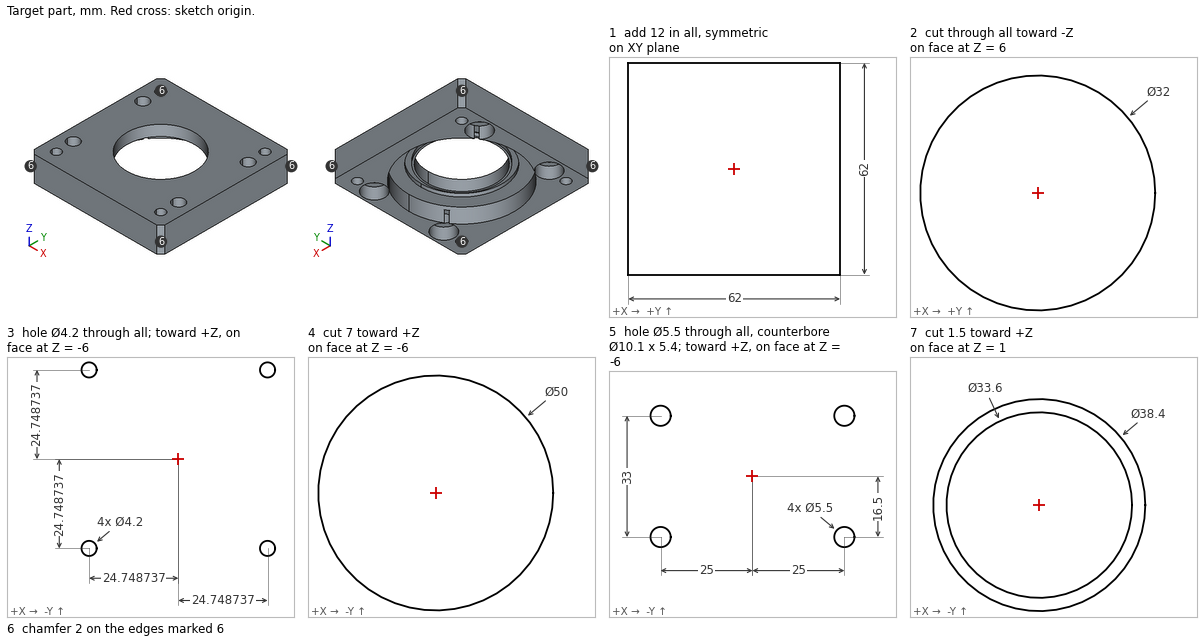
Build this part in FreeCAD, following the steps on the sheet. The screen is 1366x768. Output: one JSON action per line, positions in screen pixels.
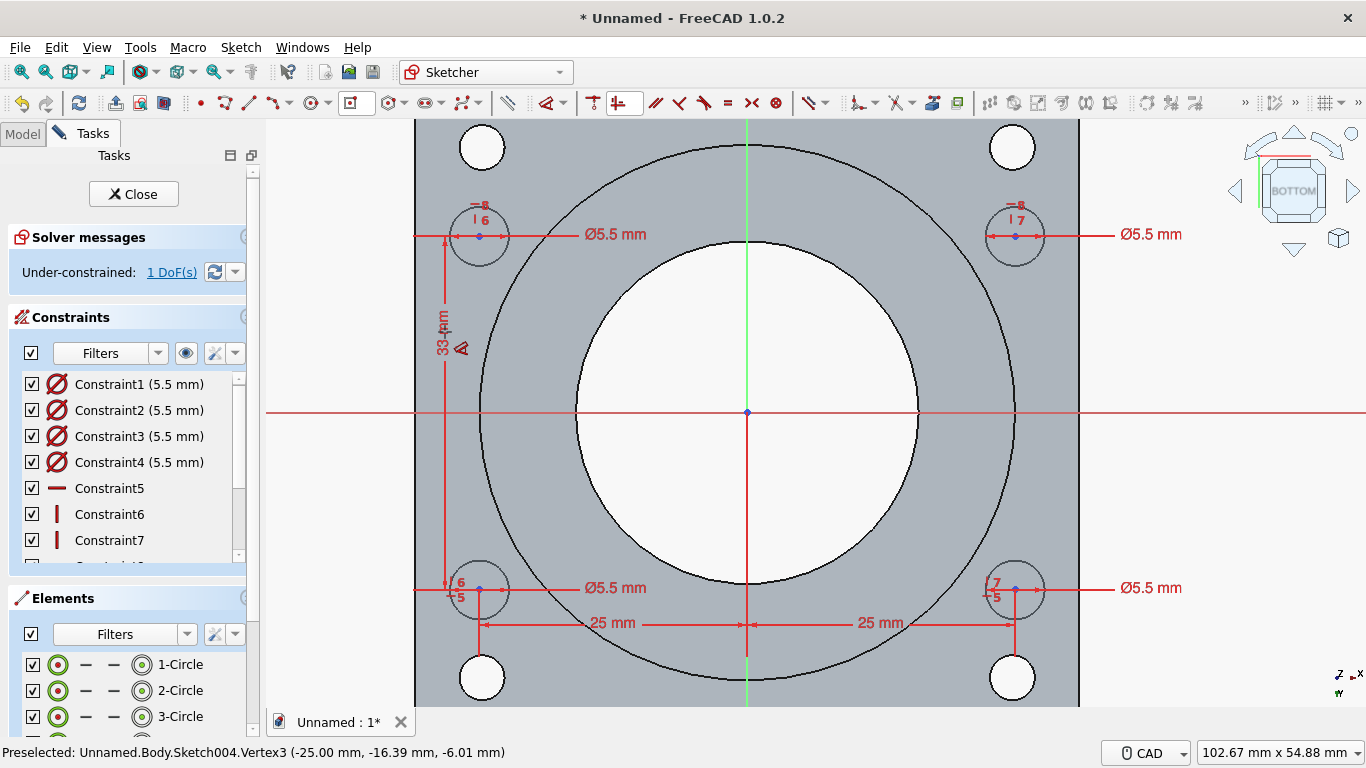
{"action": "left_click", "coordinate": [1015, 590]}
{"action": "left_click", "coordinate": [1049, 501]}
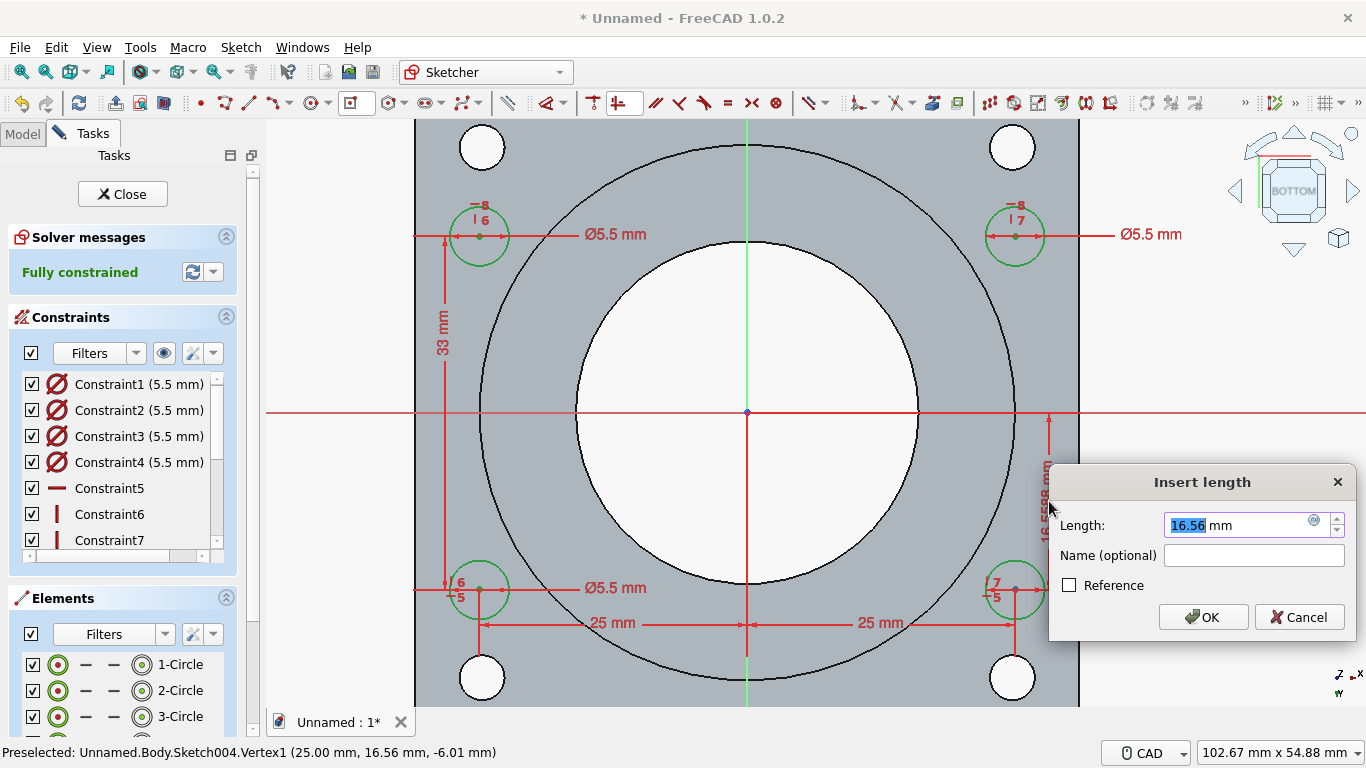
{"action": "type", "text": "16.5"}
{"action": "key", "text": "Return"}
{"action": "key", "text": "Escape"}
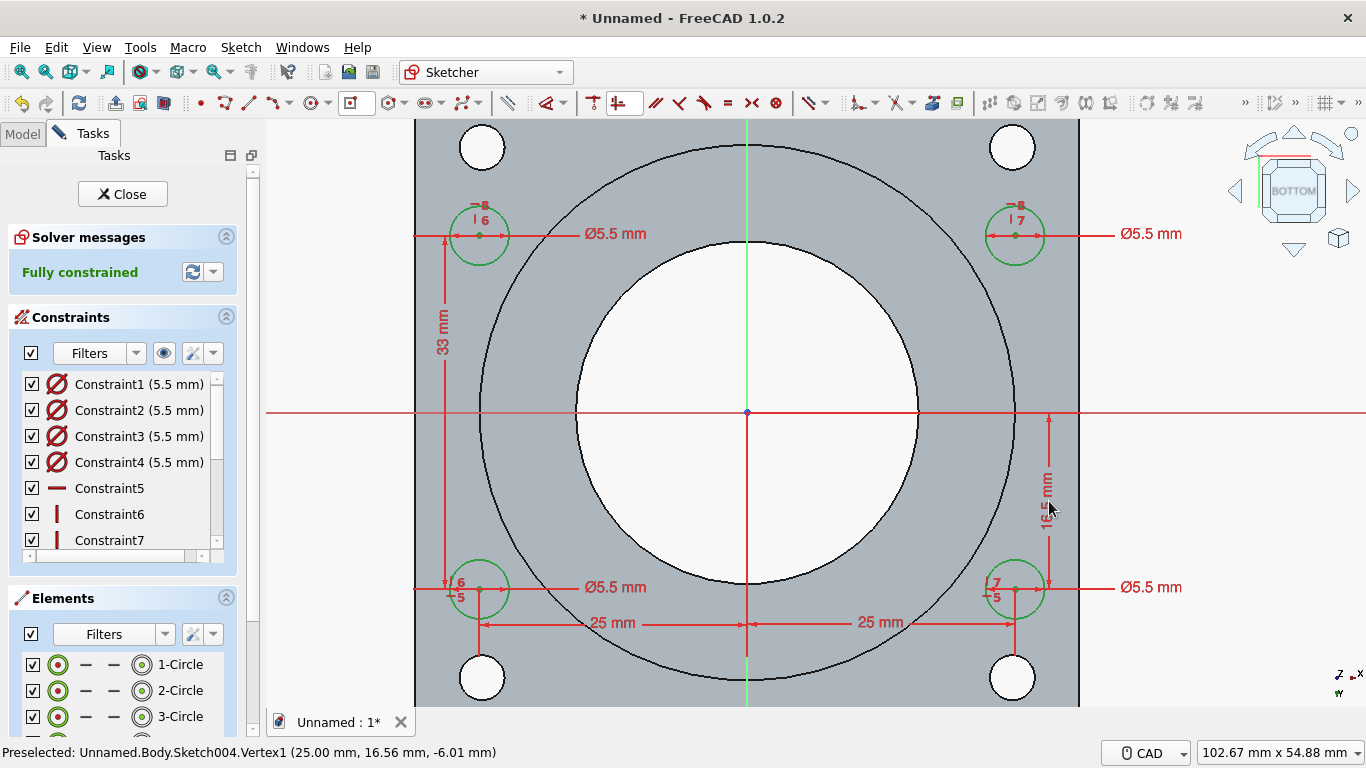
{"action": "left_click", "coordinate": [123, 194]}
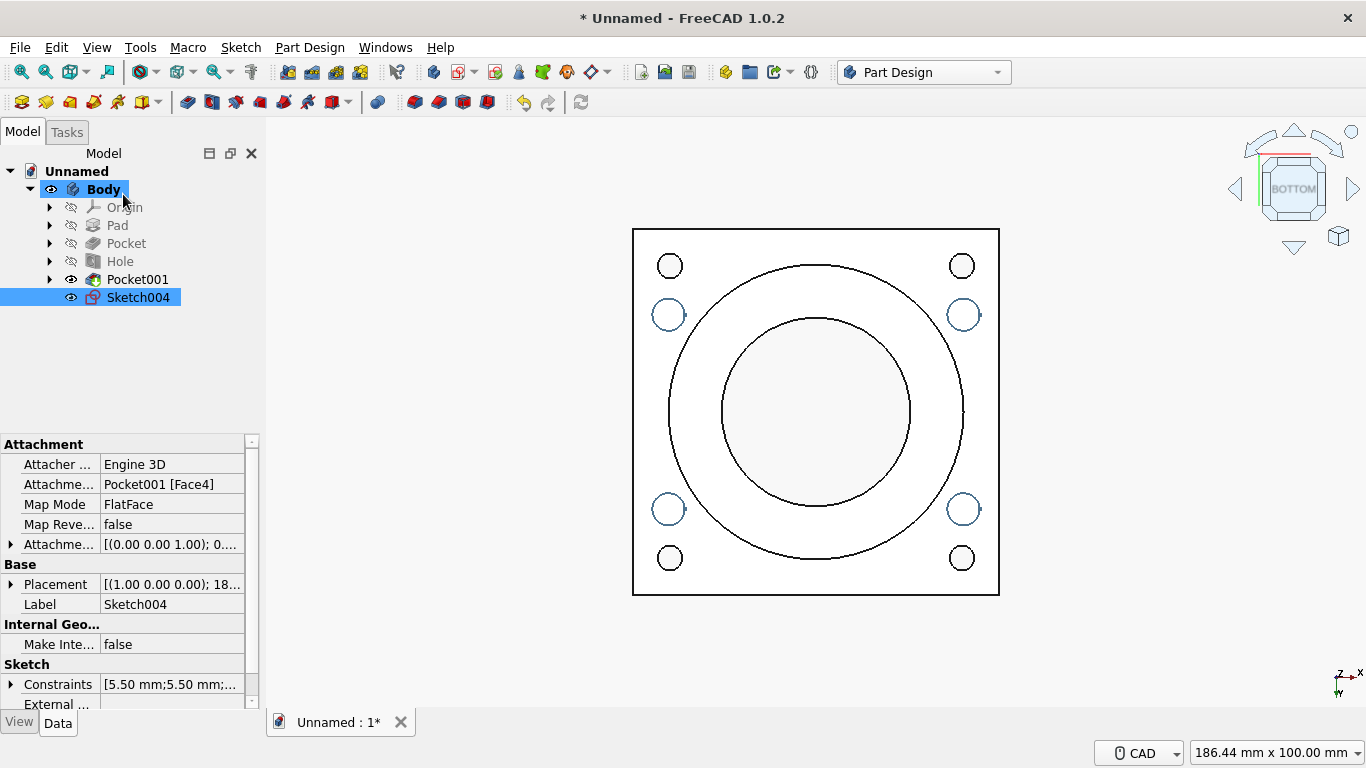
{"action": "left_click", "coordinate": [212, 102]}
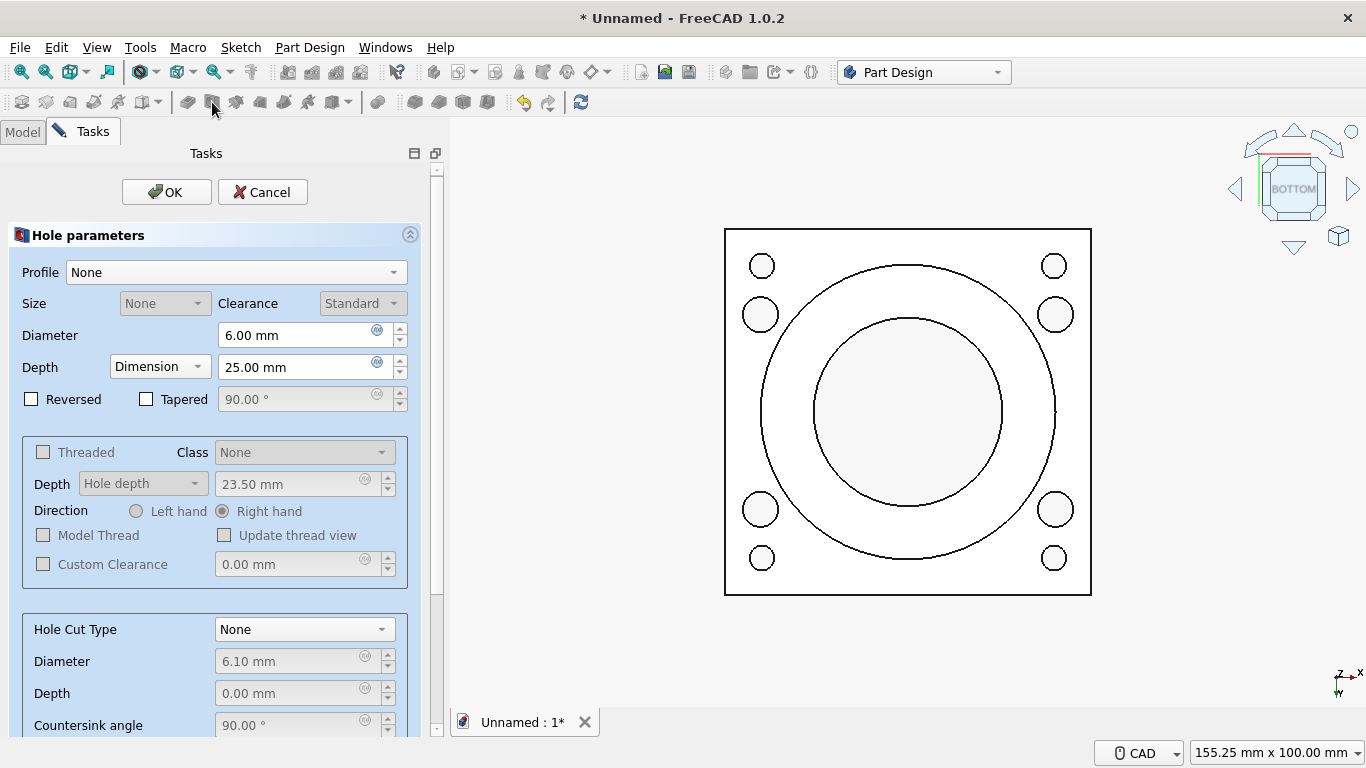
{"action": "triple_click", "coordinate": [305, 335]}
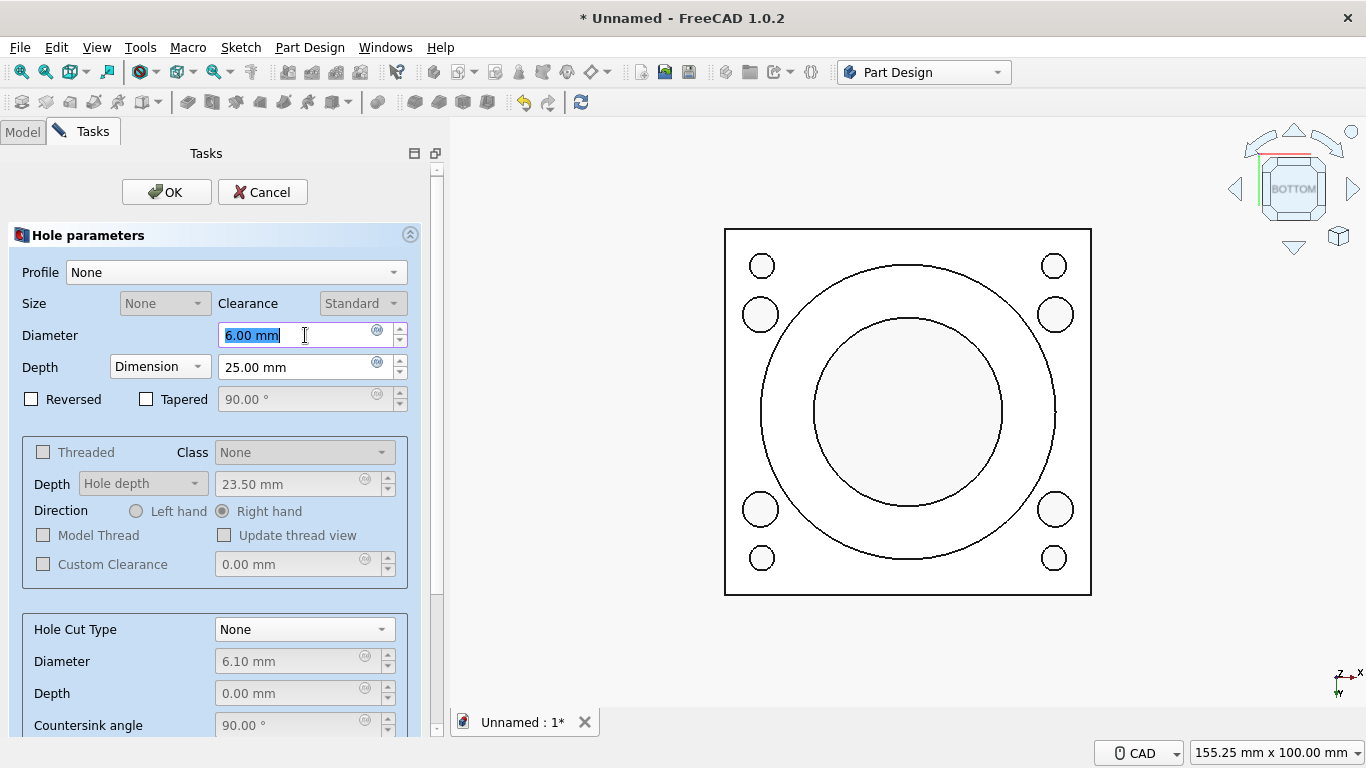
{"action": "type", "text": "5.5"}
{"action": "key", "text": "Tab"}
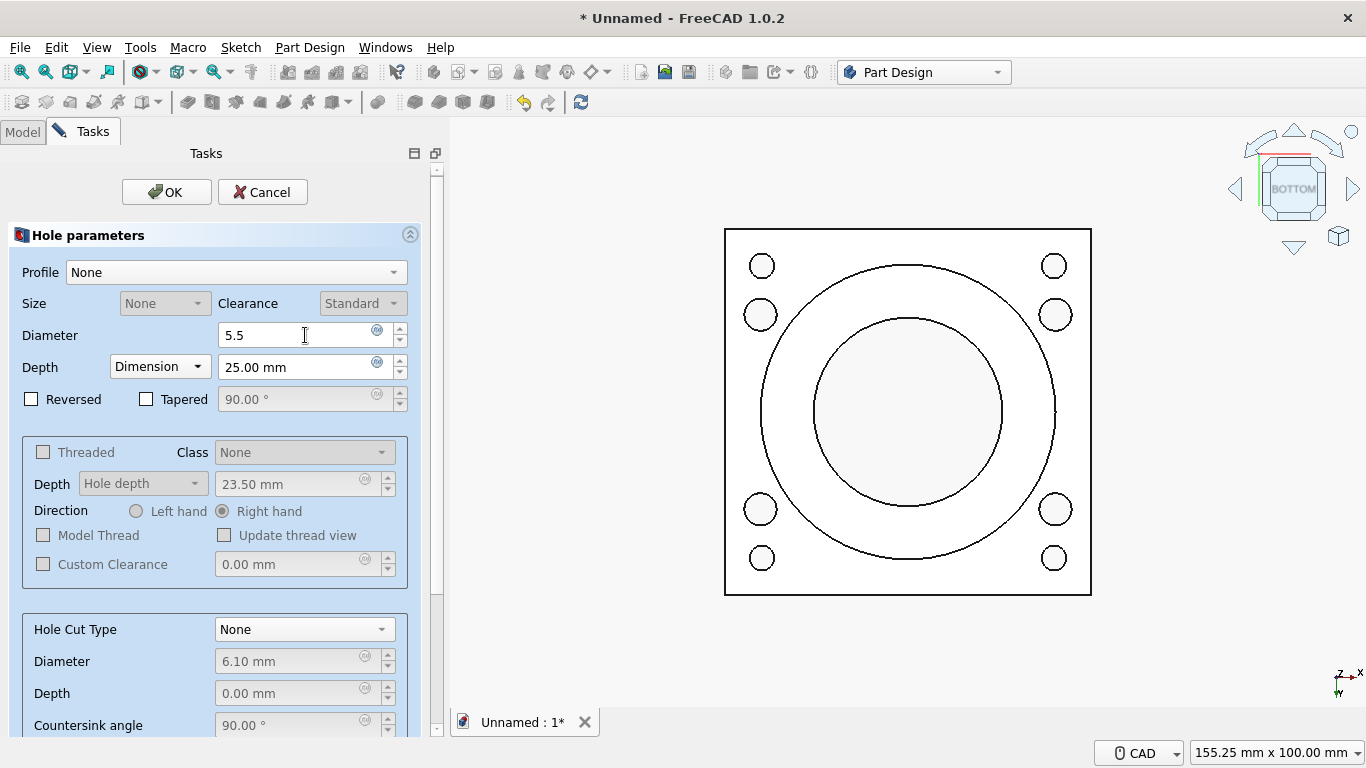
{"action": "left_click", "coordinate": [161, 366]}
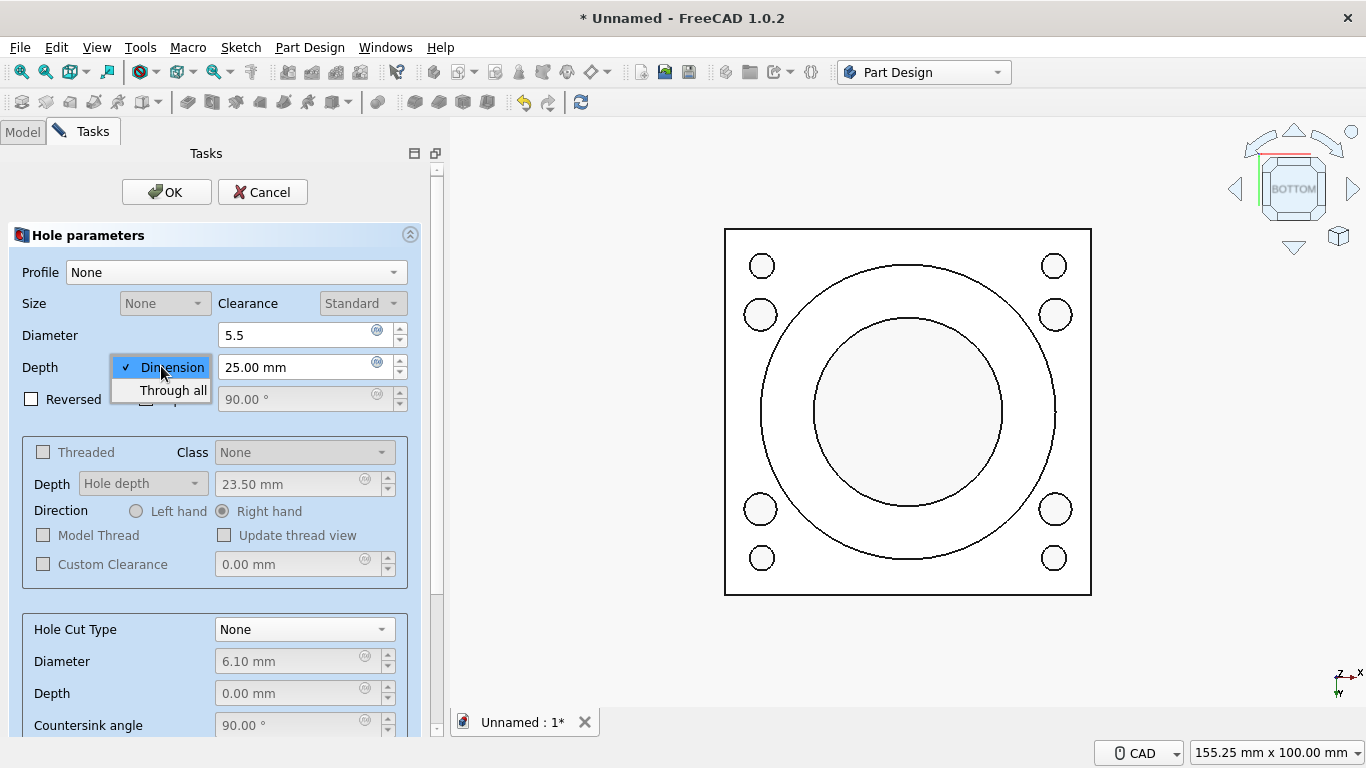
{"action": "left_click", "coordinate": [160, 390]}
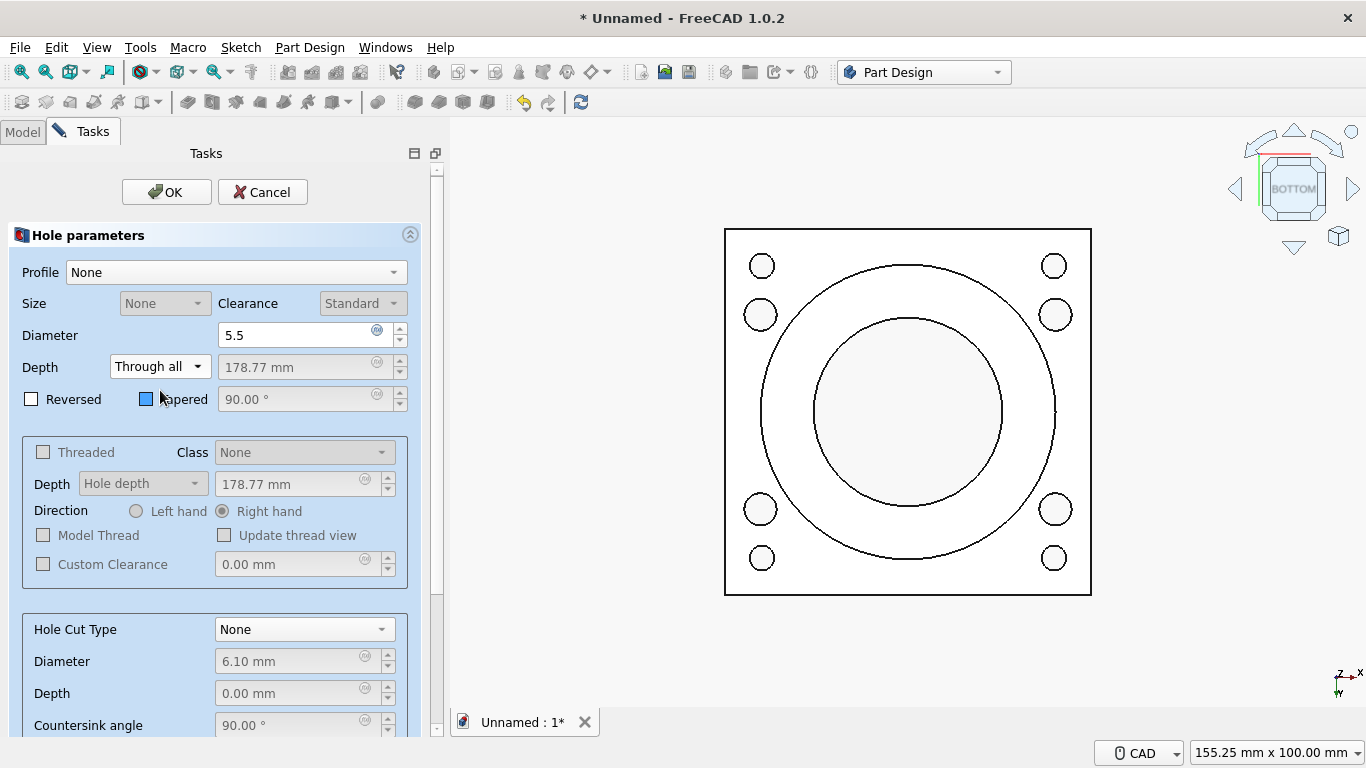
{"action": "left_click", "coordinate": [306, 630]}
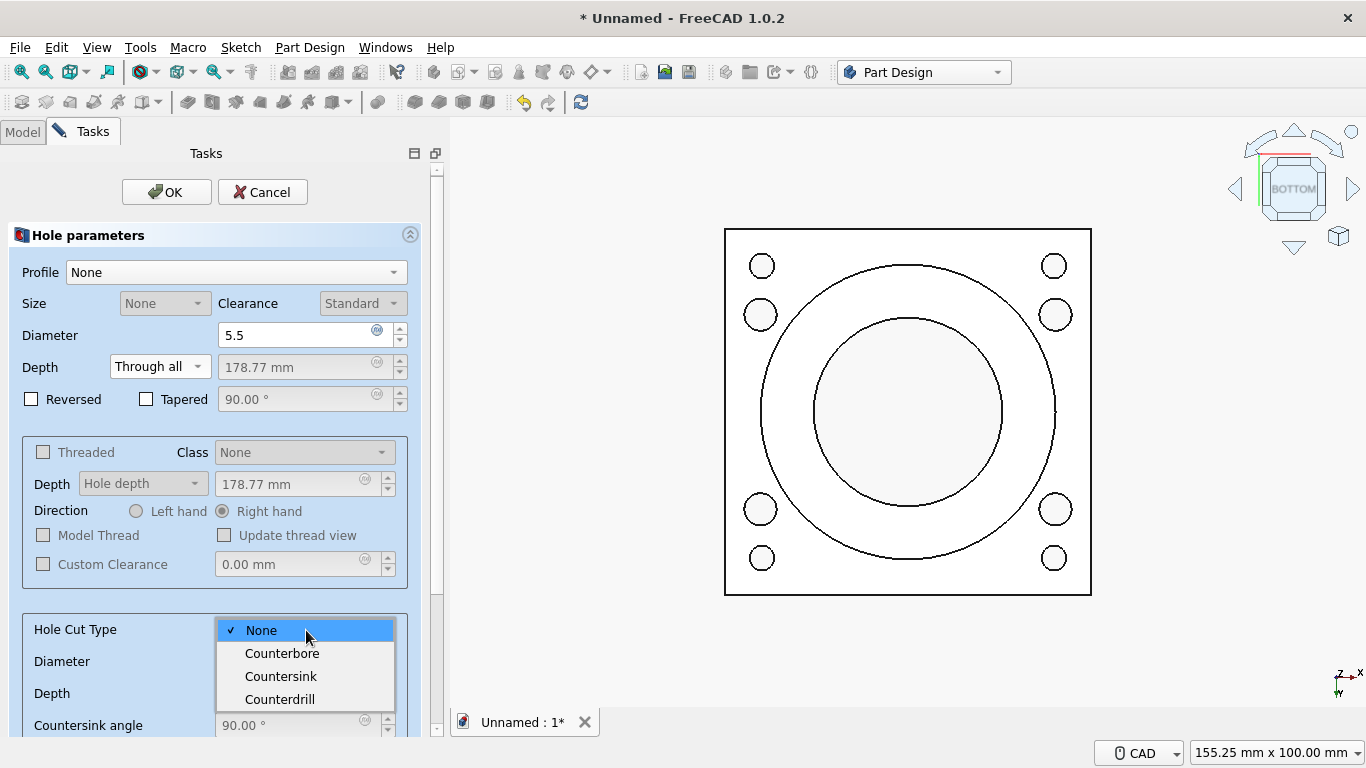
{"action": "left_click", "coordinate": [304, 654]}